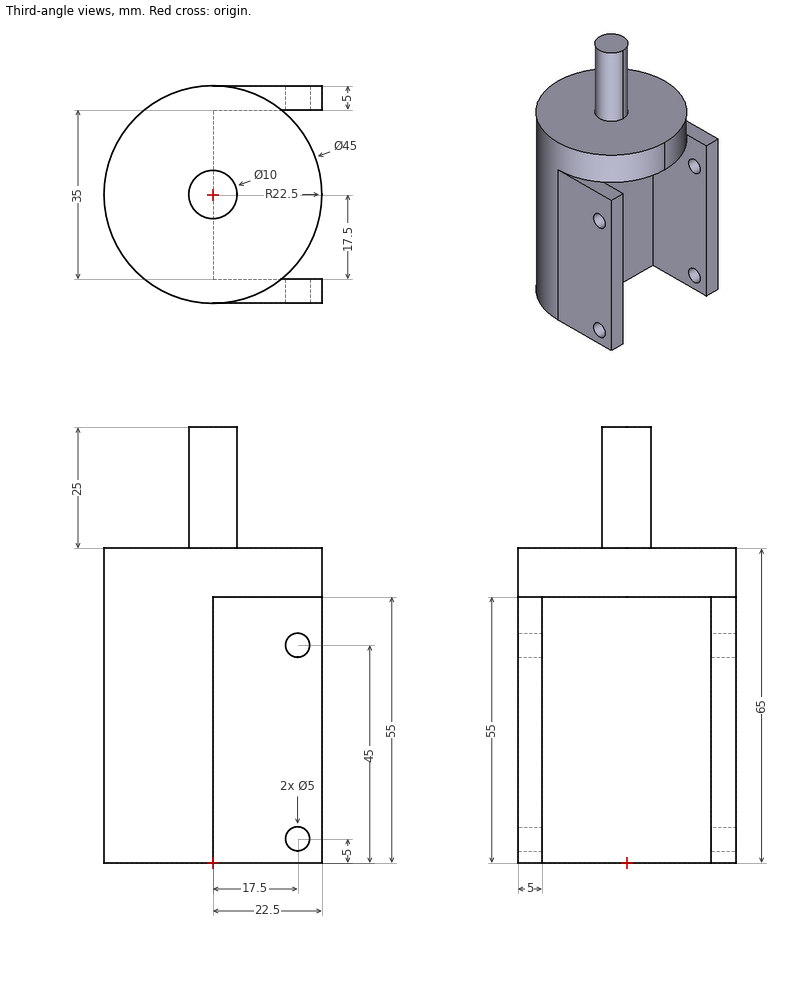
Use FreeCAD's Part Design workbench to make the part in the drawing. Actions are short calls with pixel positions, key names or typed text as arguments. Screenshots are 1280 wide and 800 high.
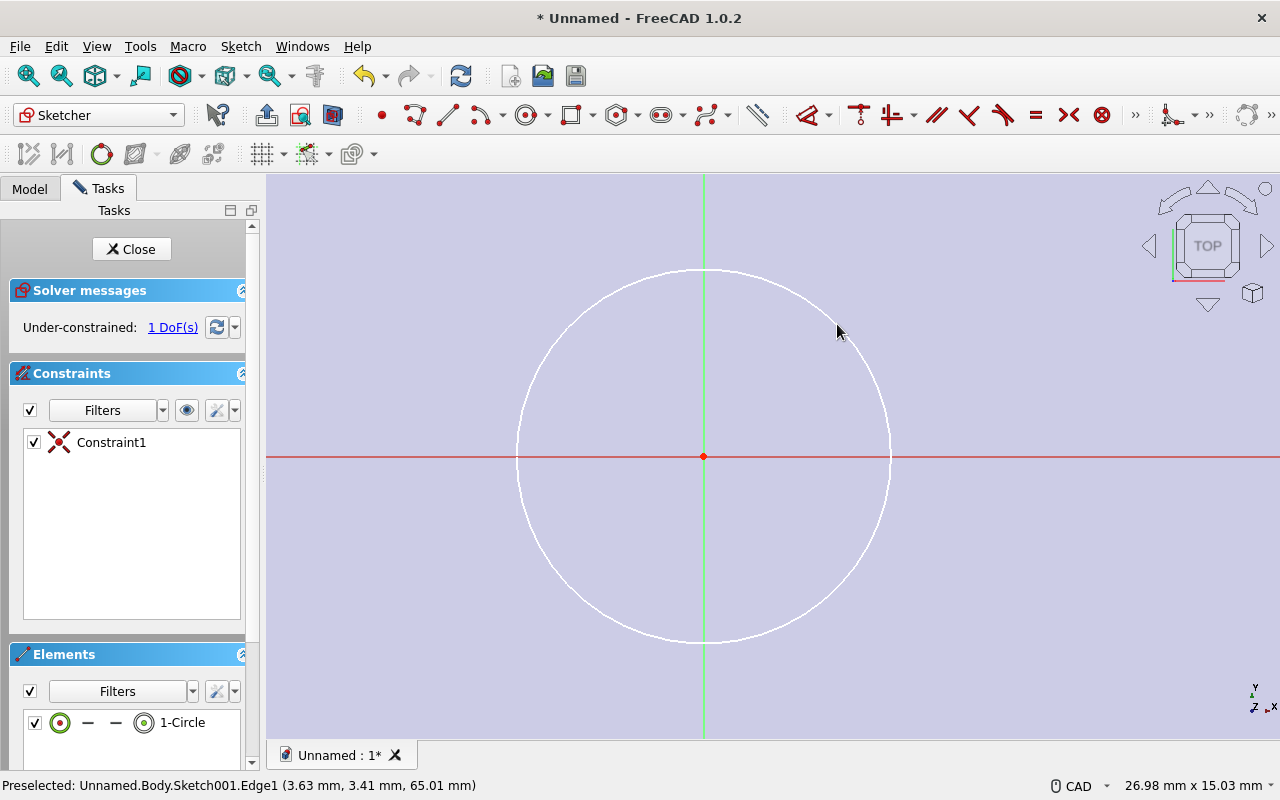
click(806, 116)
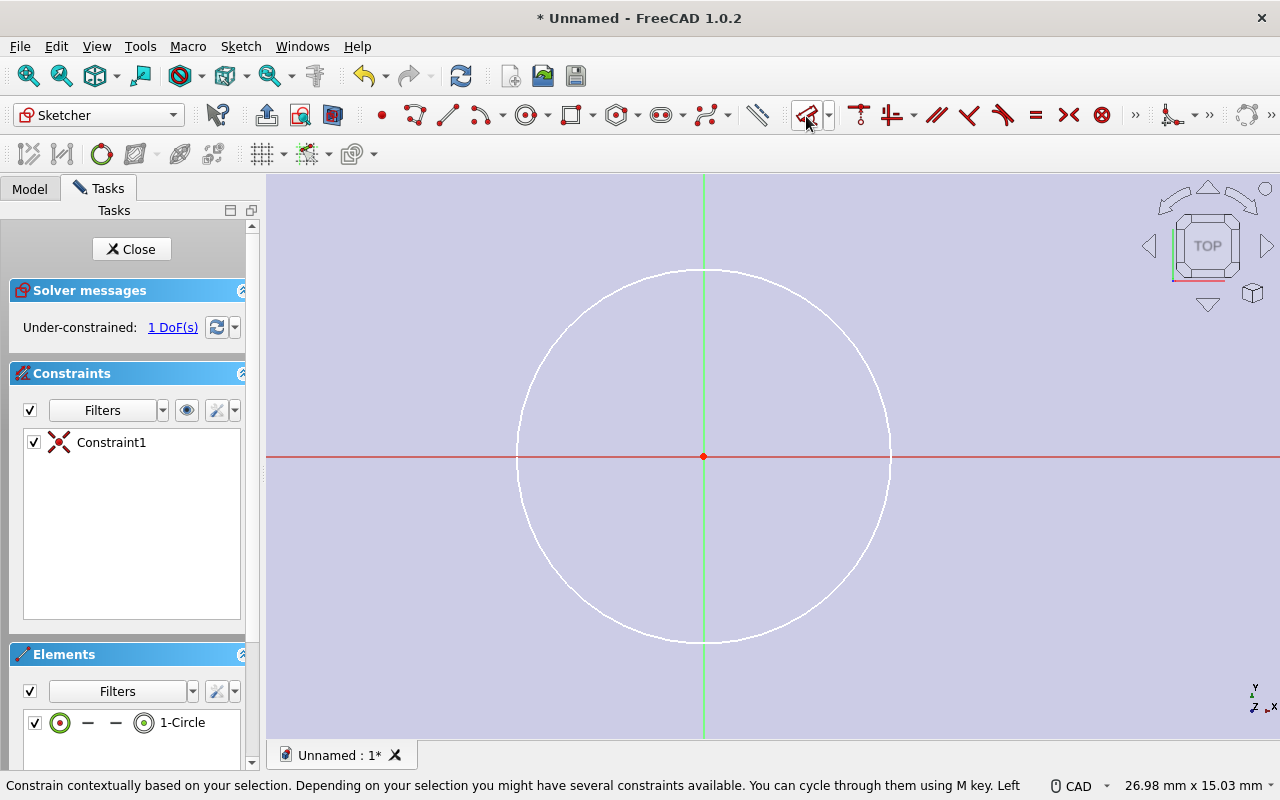
click(836, 324)
click(859, 301)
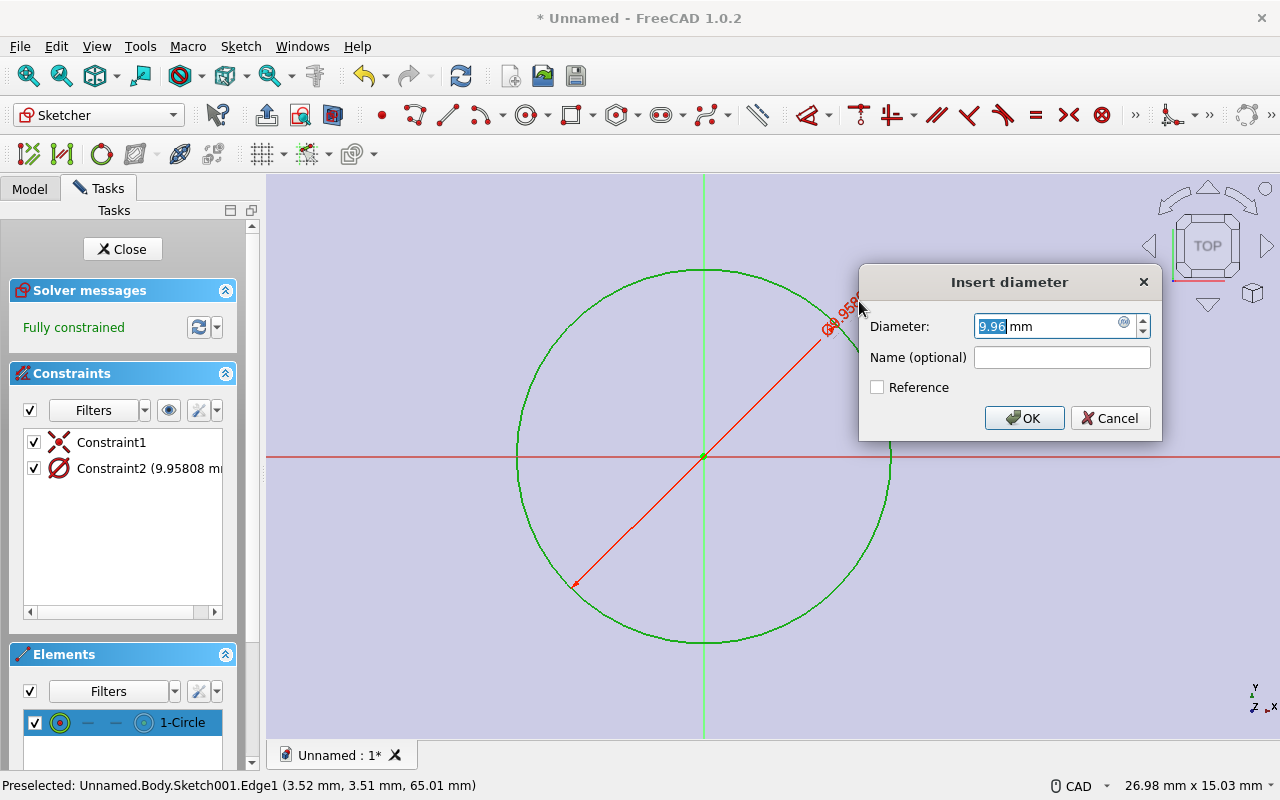
text(10)
key(Return)
key(Escape)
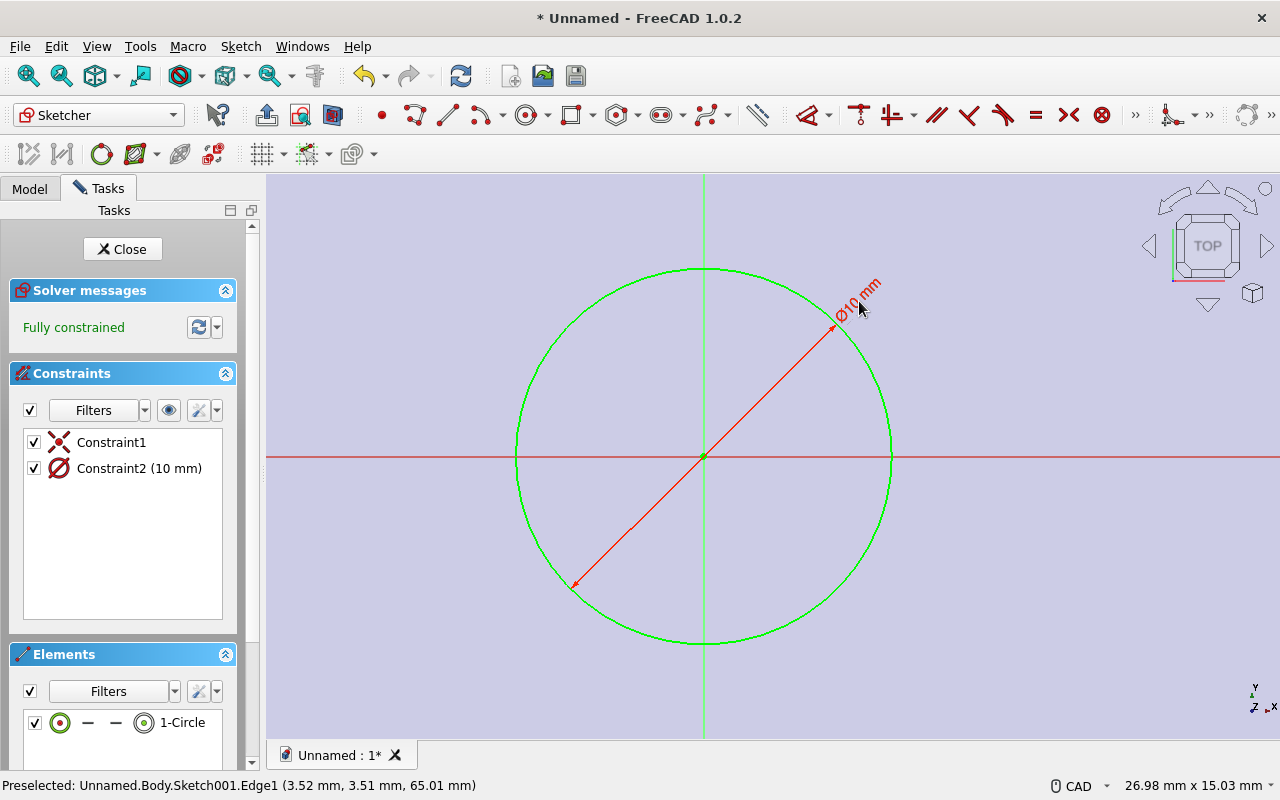
click(123, 249)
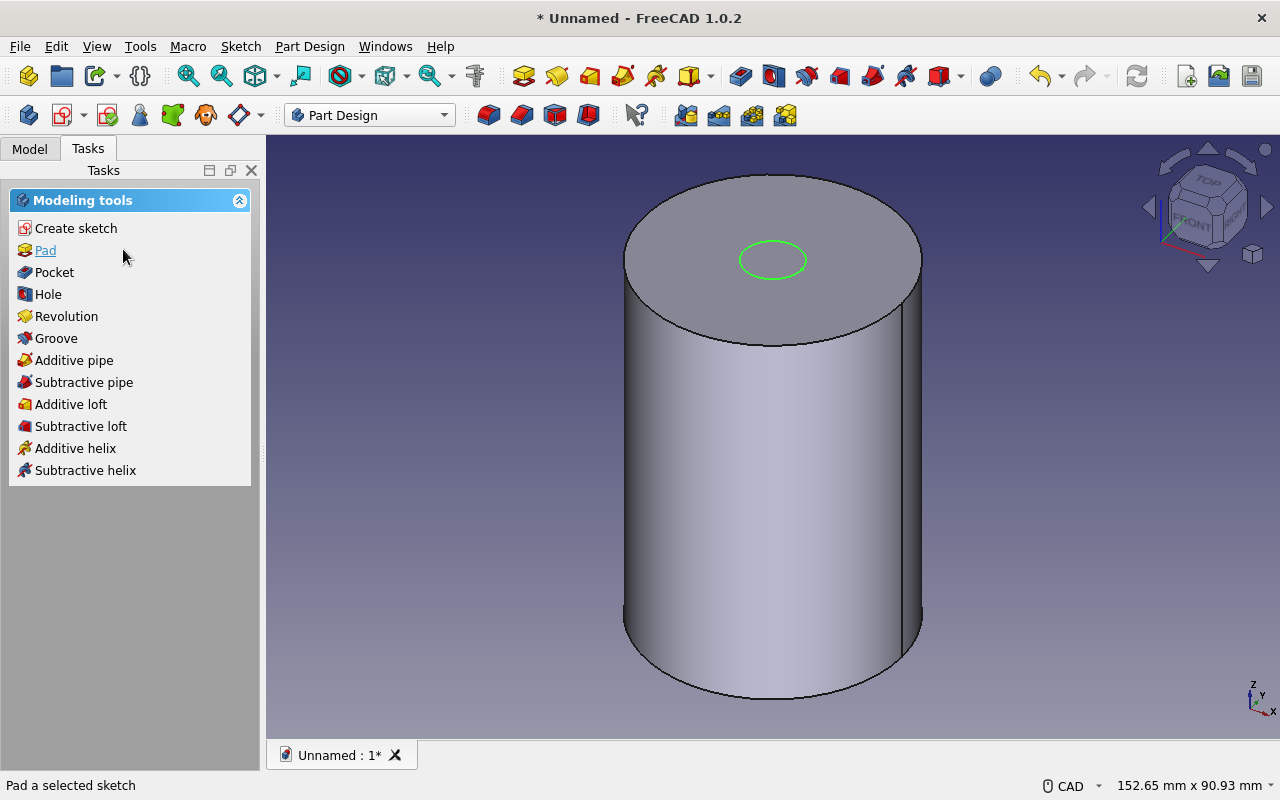
click(524, 76)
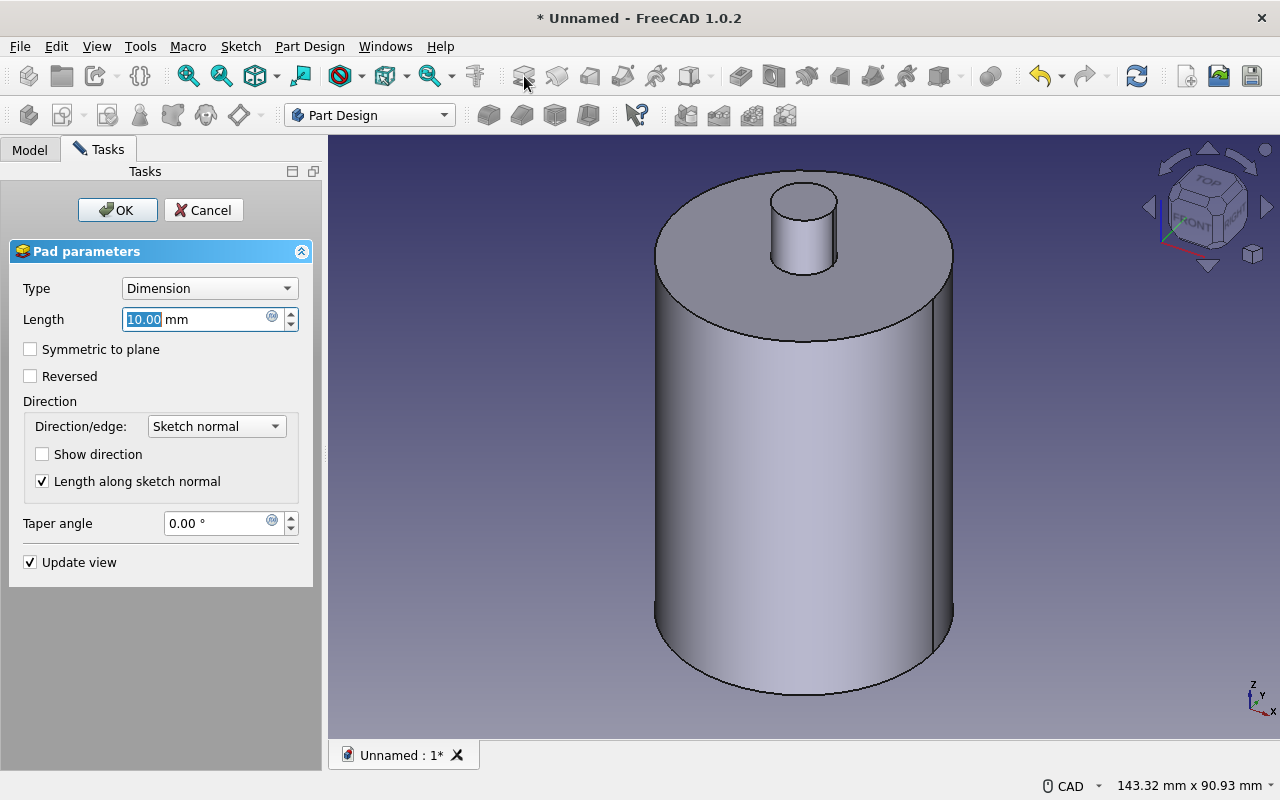
text(25)
key(Tab)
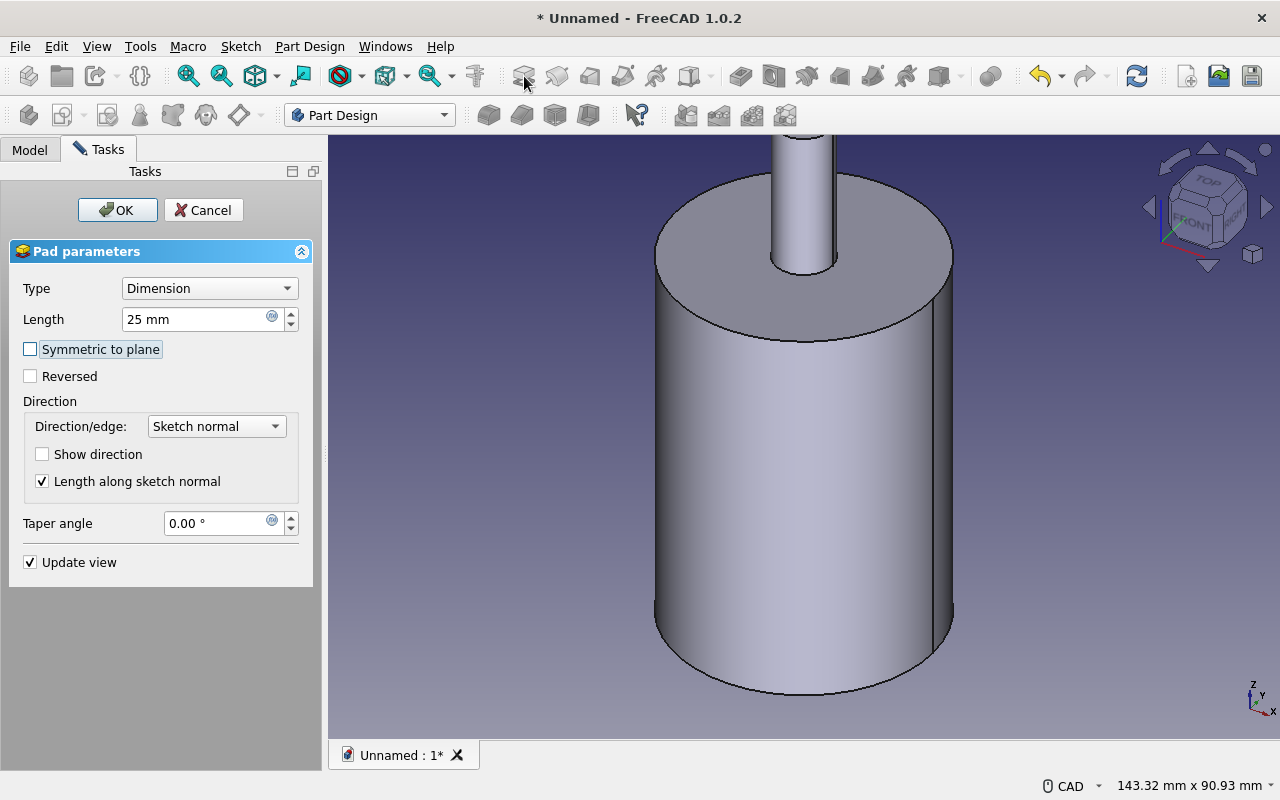
click(118, 210)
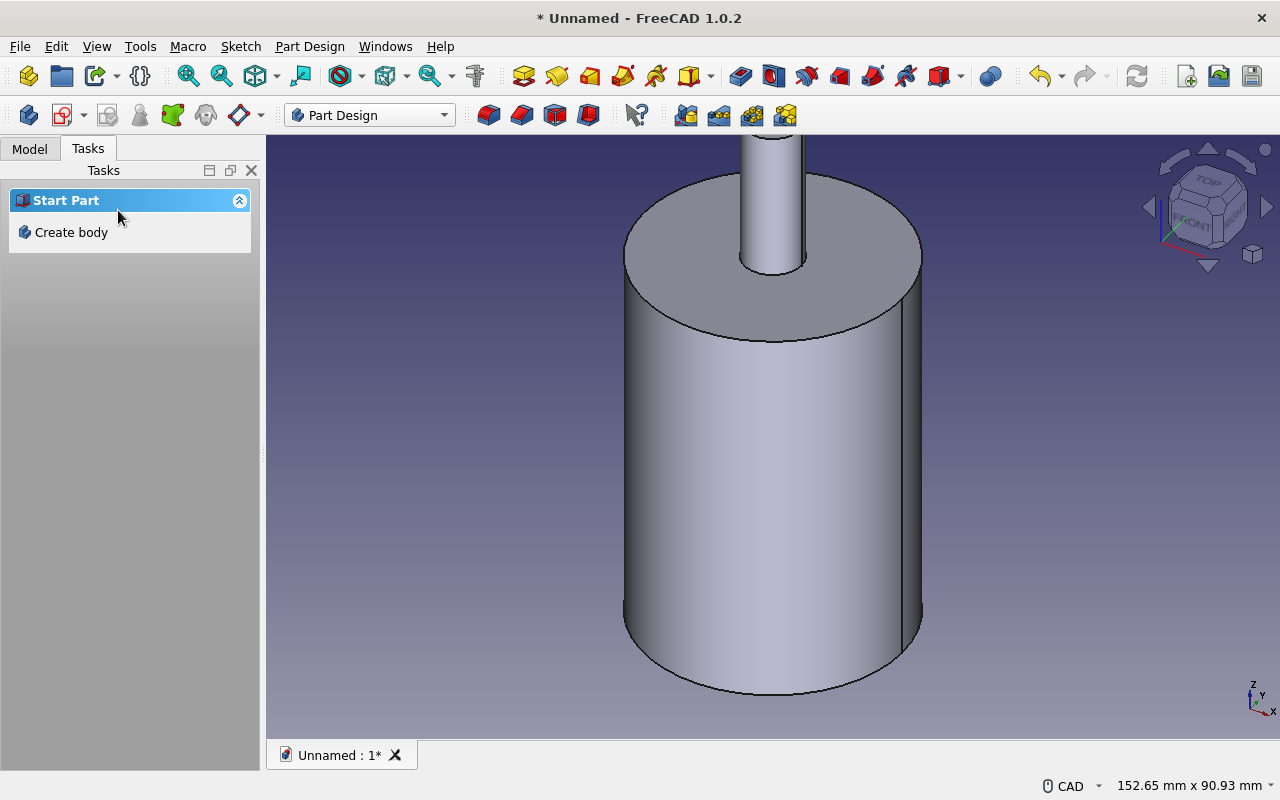
click(189, 76)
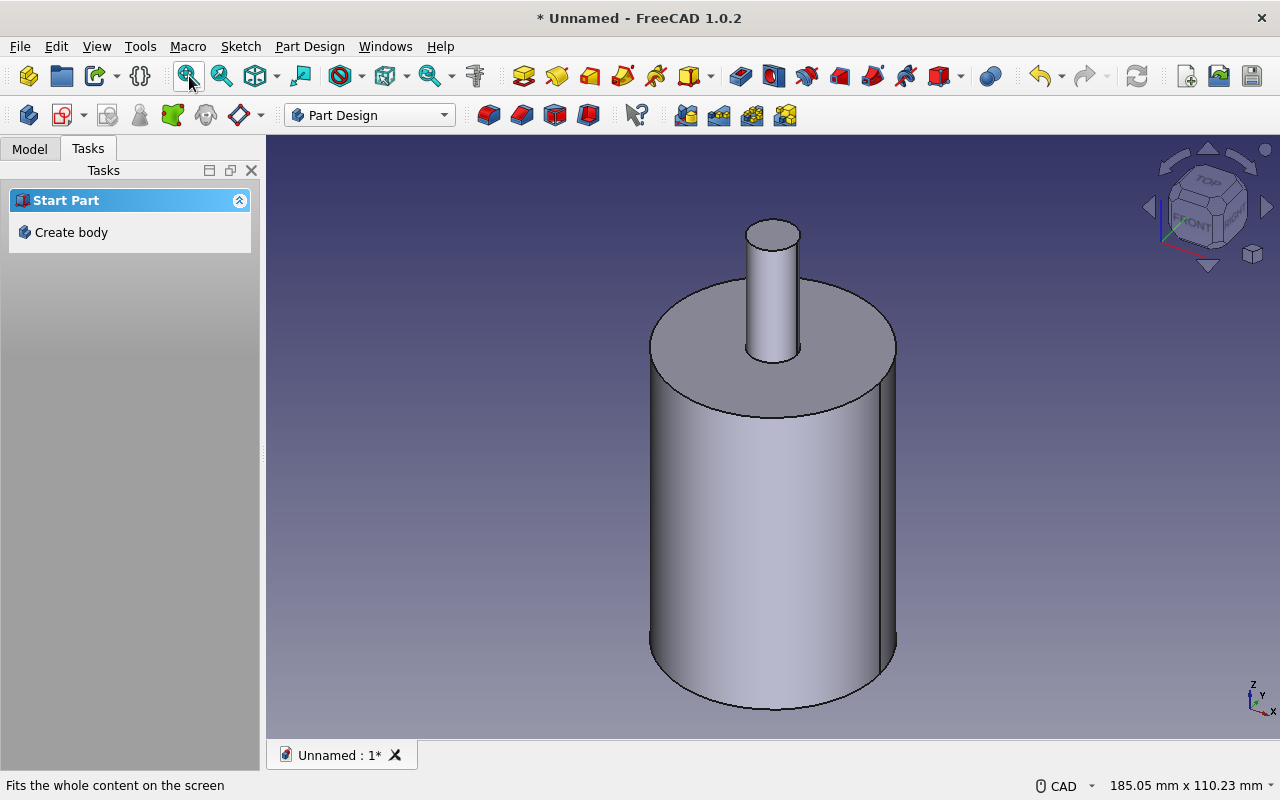
click(30, 148)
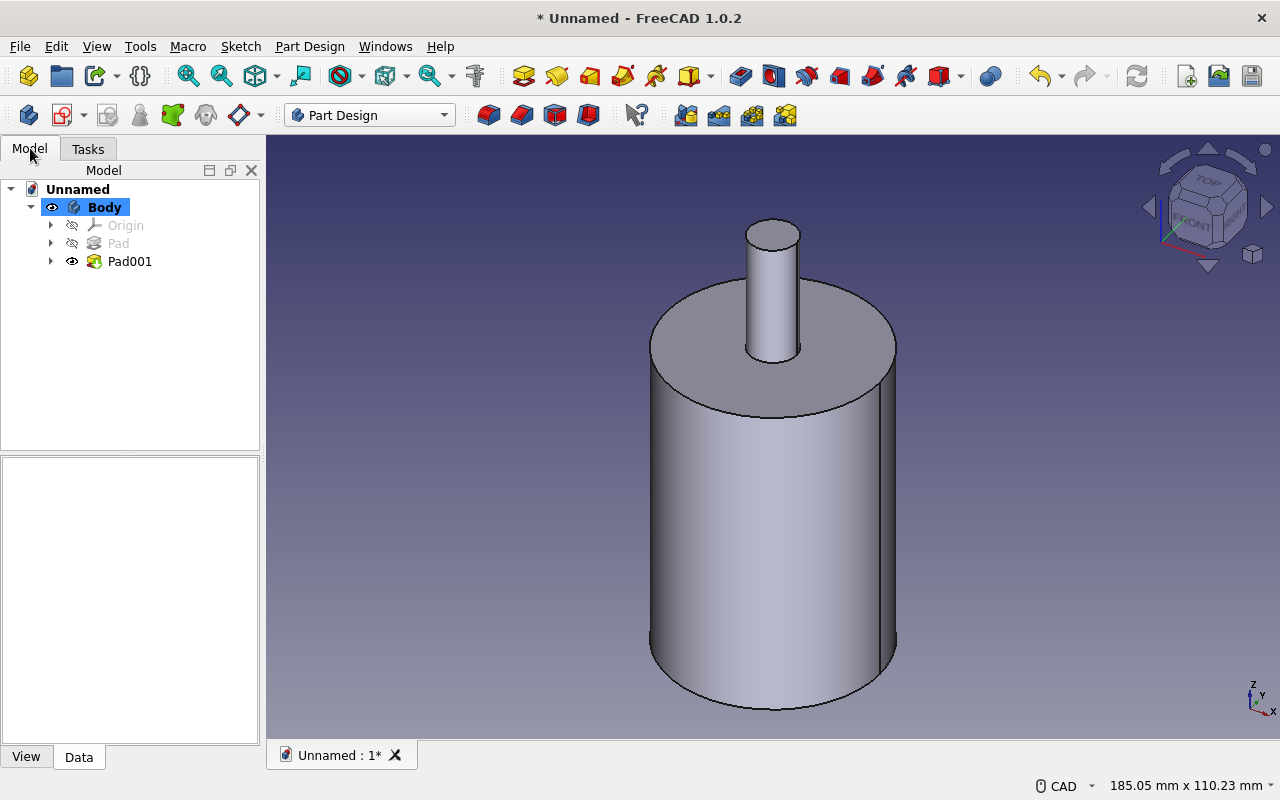
click(51, 225)